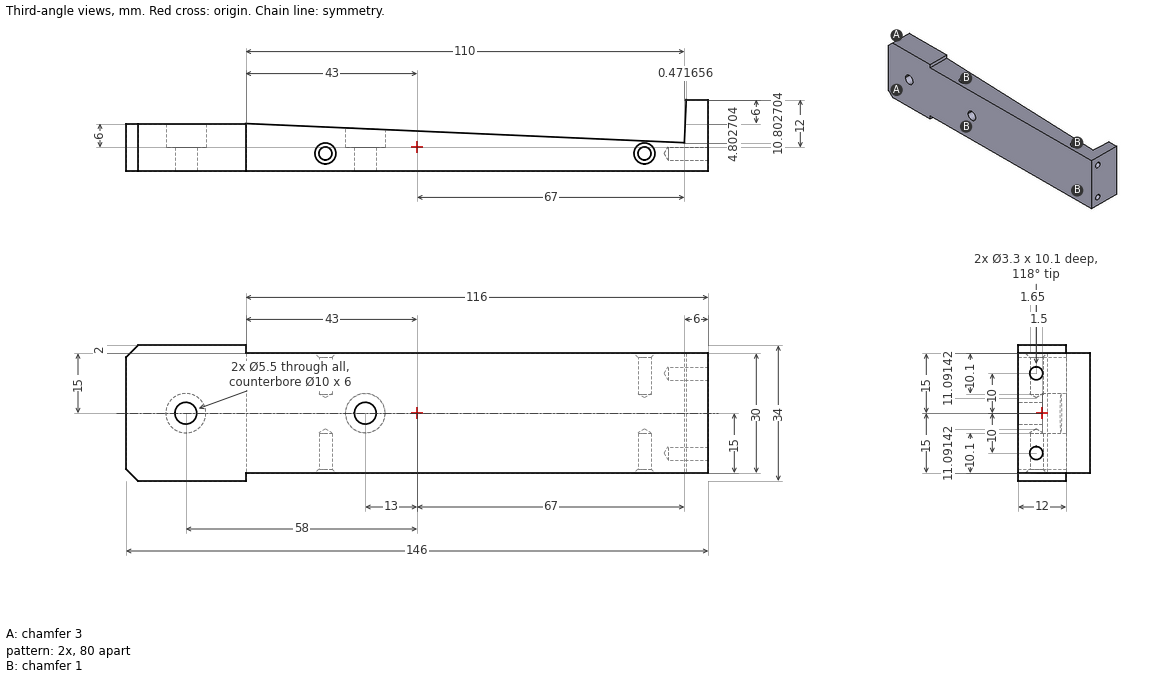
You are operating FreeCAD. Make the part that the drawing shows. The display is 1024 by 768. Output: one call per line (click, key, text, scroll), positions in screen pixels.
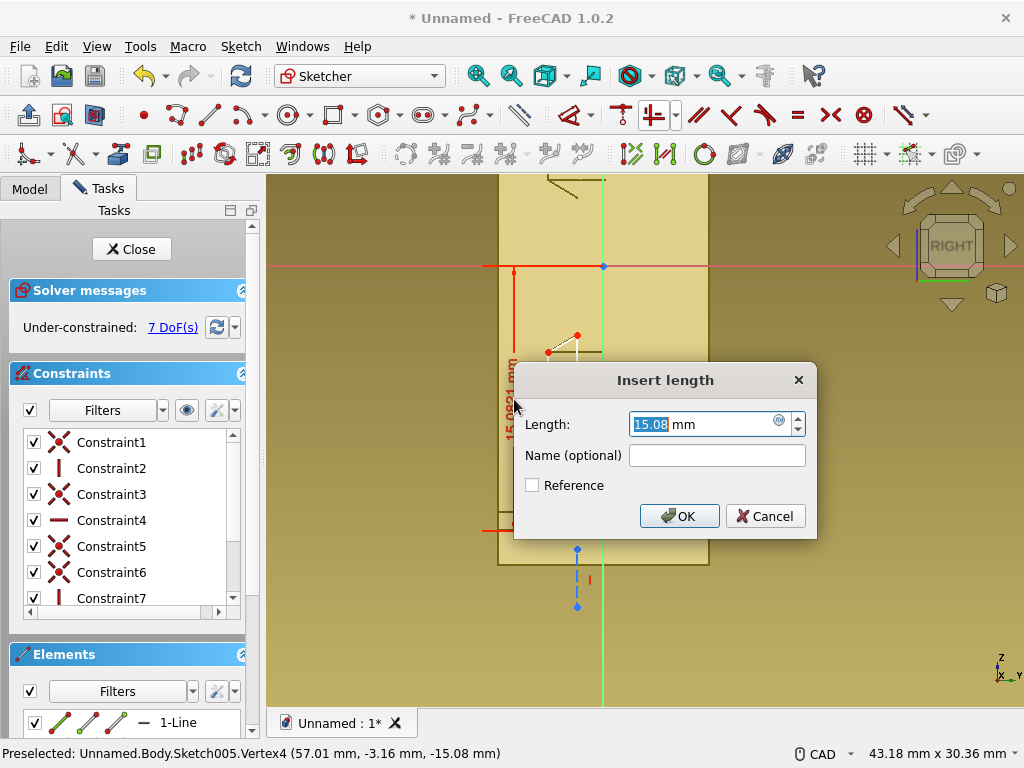
text(15)
key(Return)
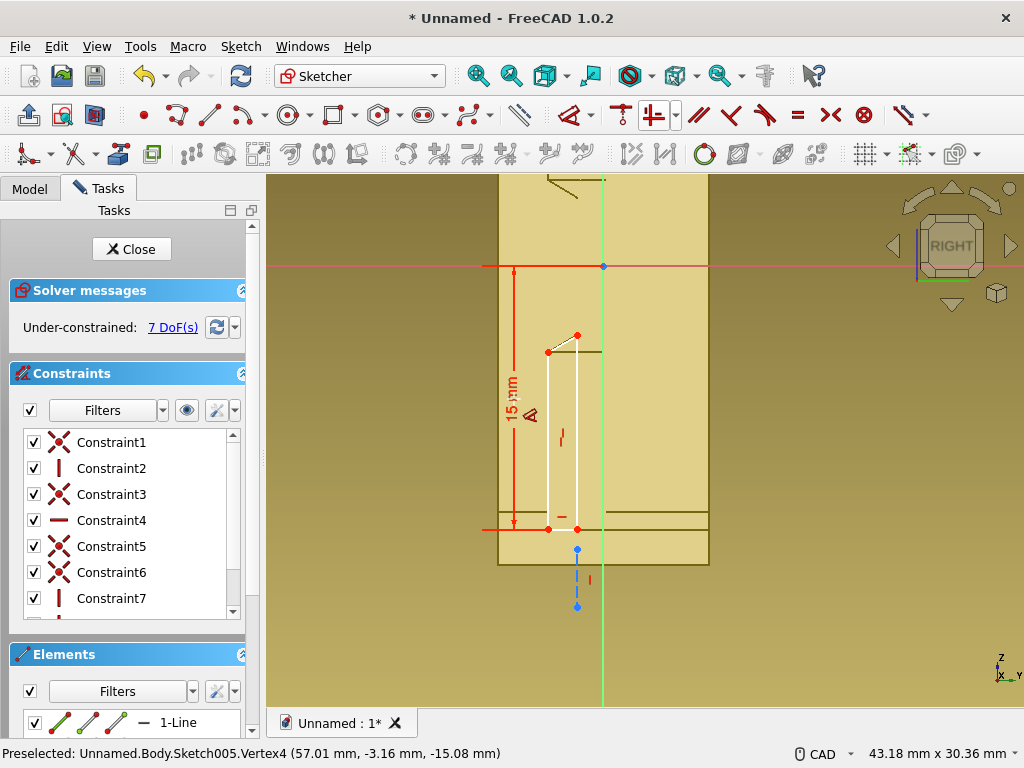
click(548, 406)
click(514, 441)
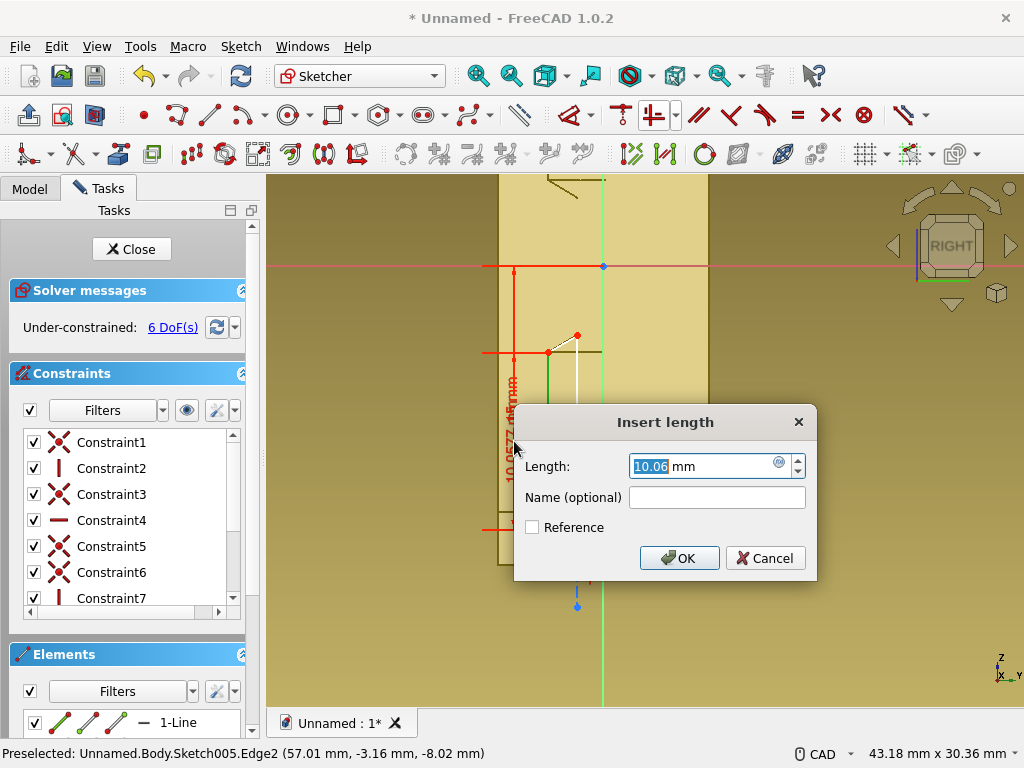
text(10.1)
key(Return)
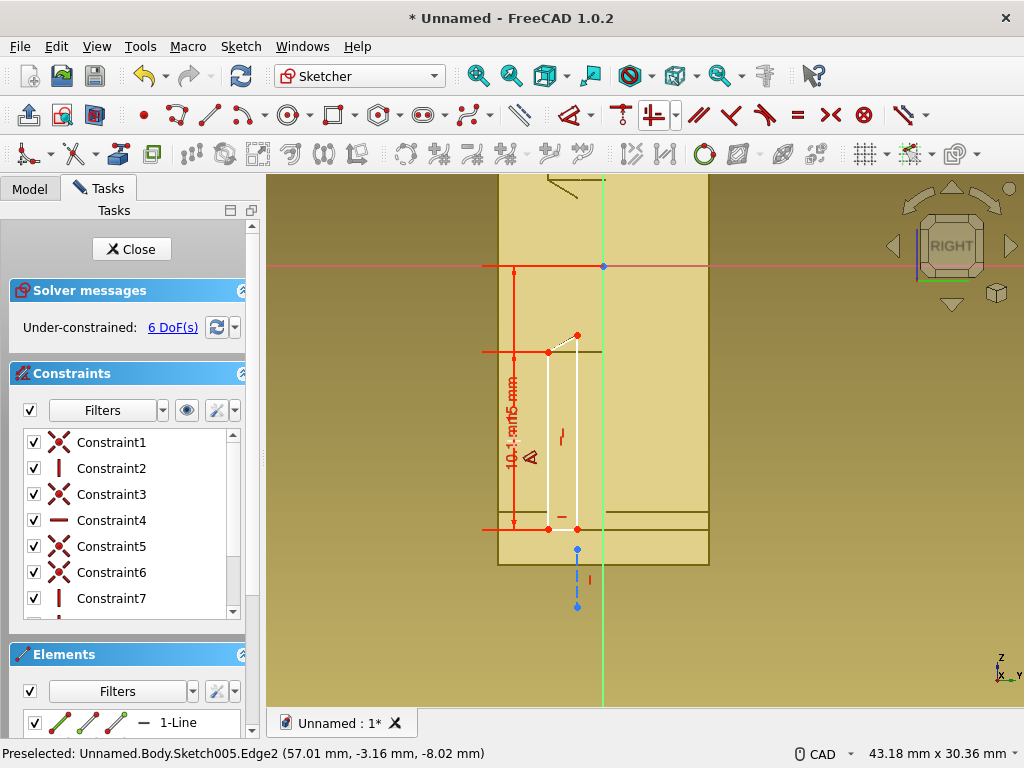
scroll(560, 530, up, 2)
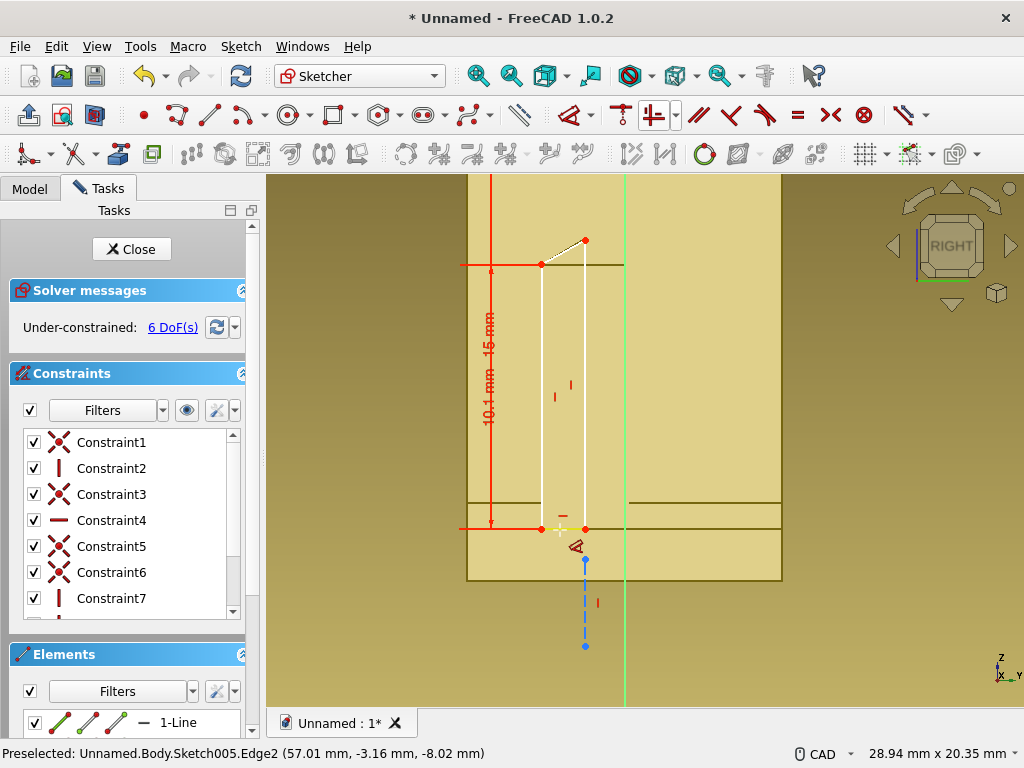
click(559, 529)
click(564, 563)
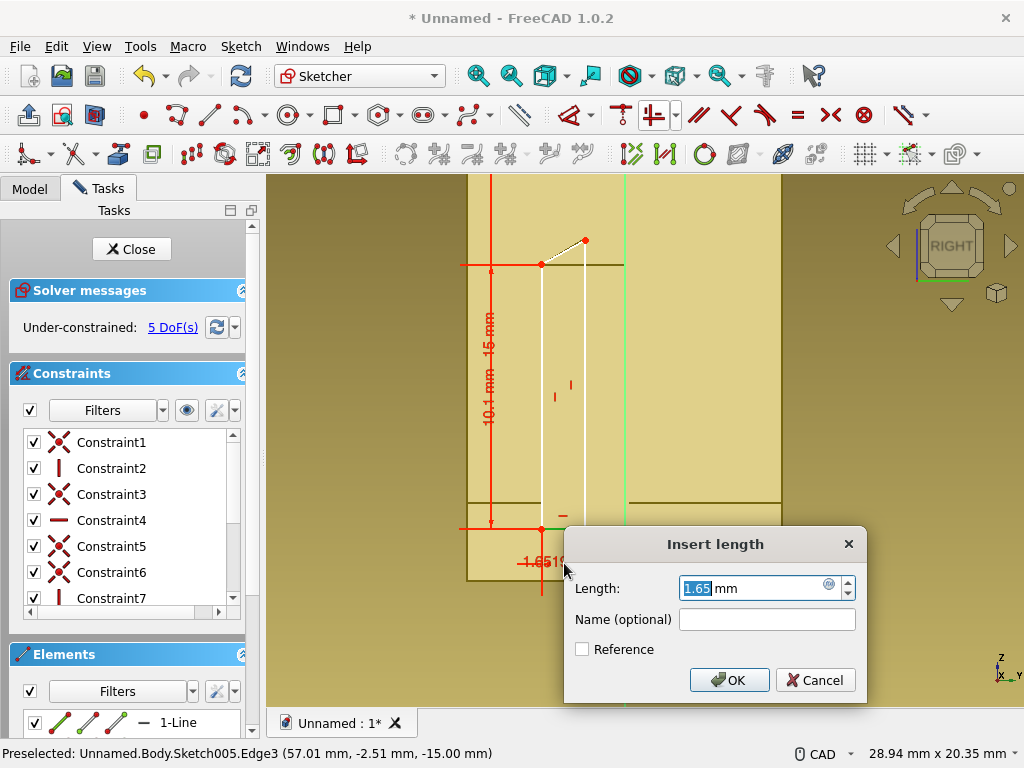
text(1.65)
key(Return)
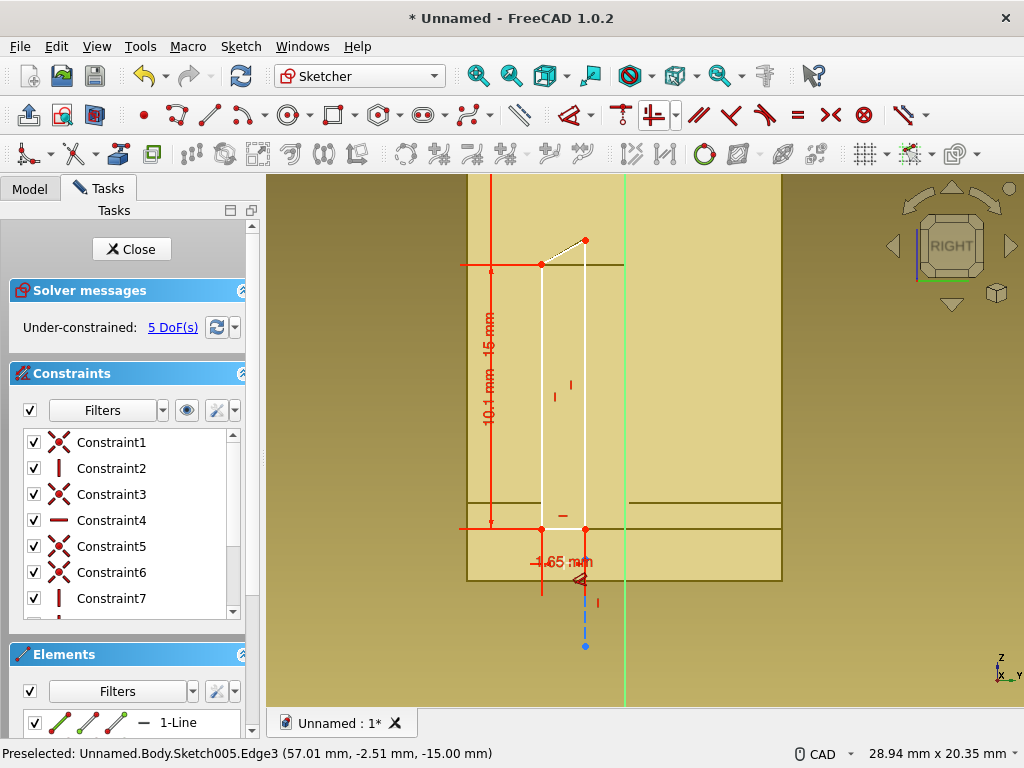
click(585, 240)
click(605, 274)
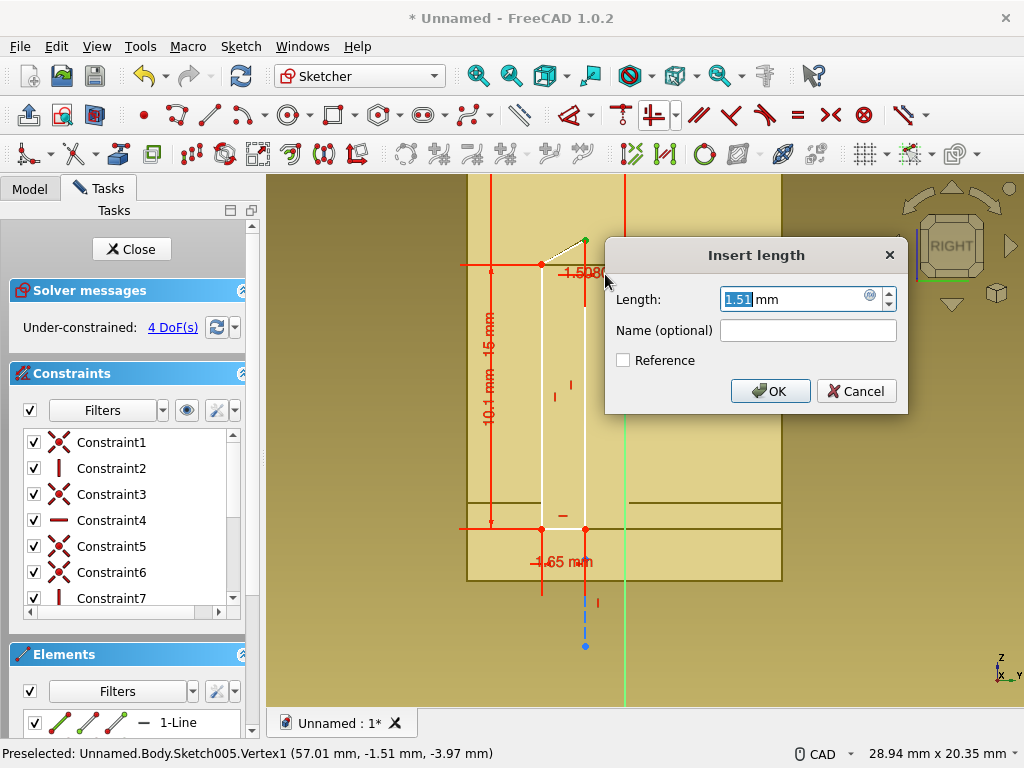
text(1.5)
key(Return)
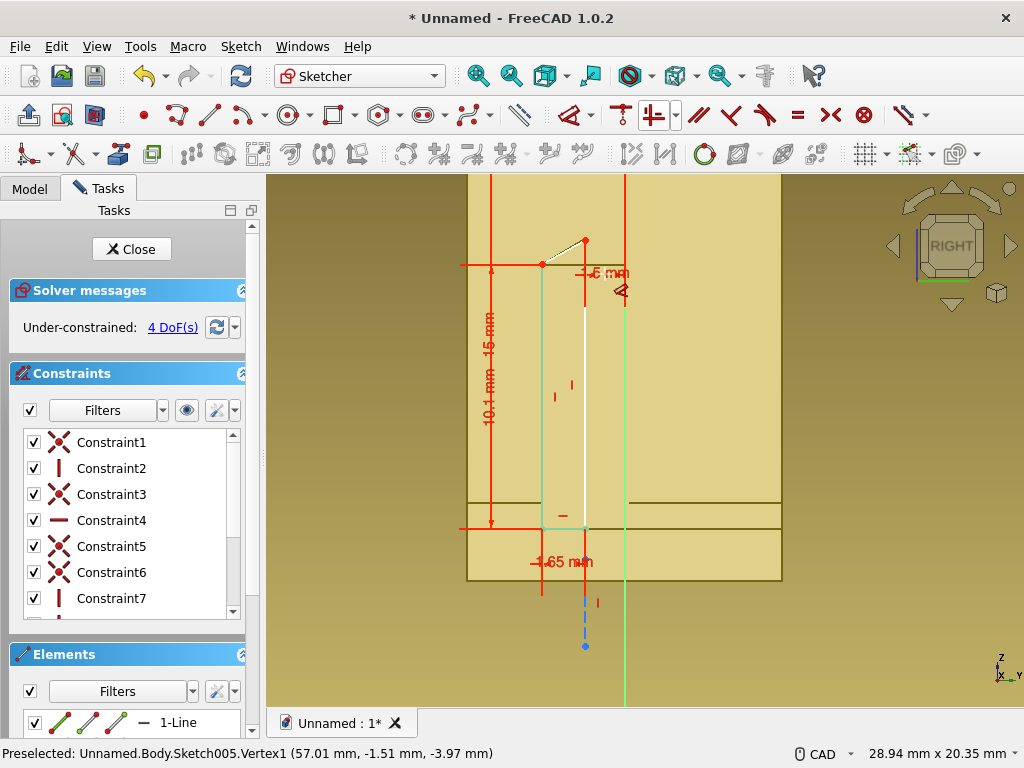
click(585, 560)
click(605, 594)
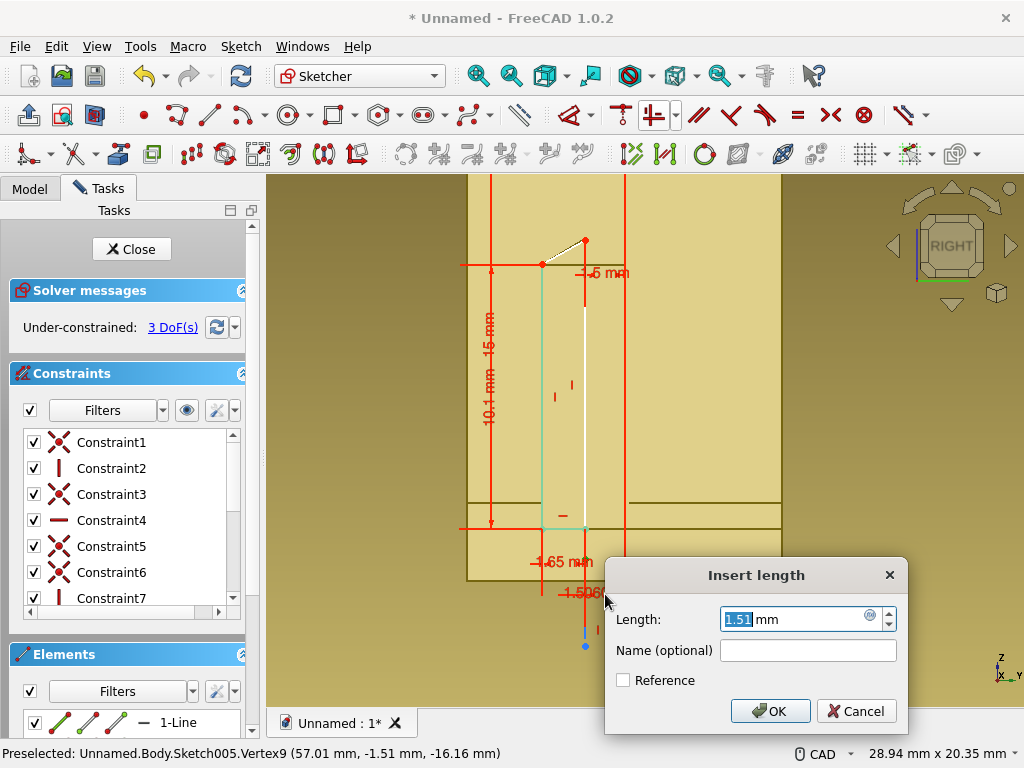
text(1.5)
key(Return)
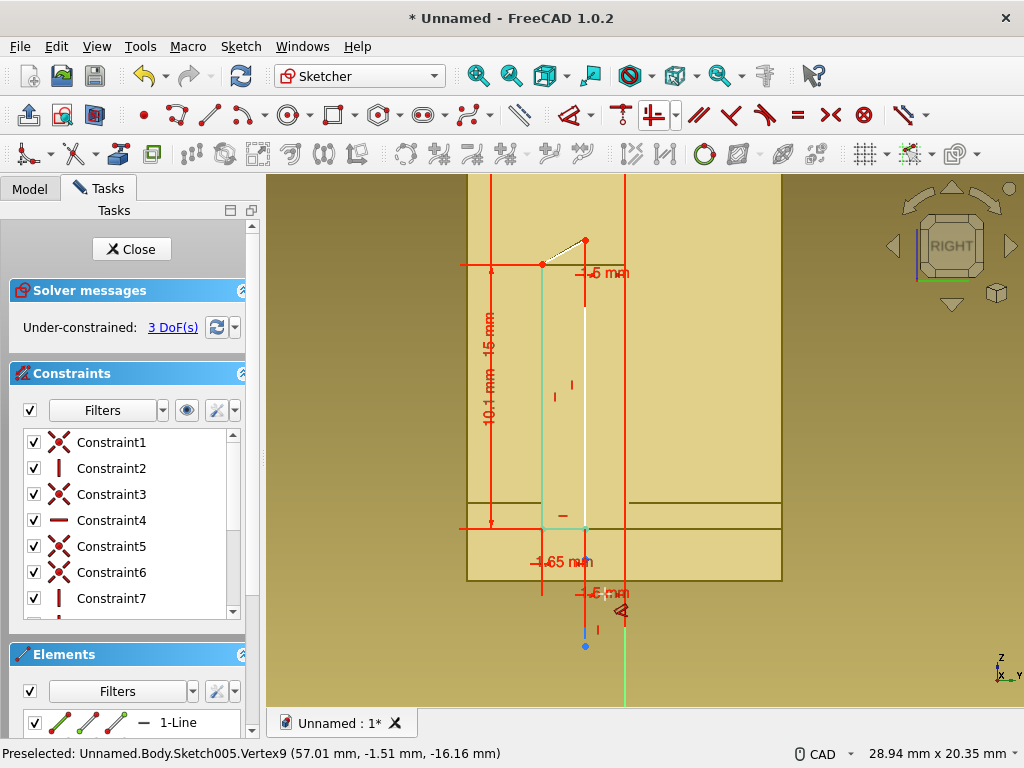
click(585, 442)
click(643, 385)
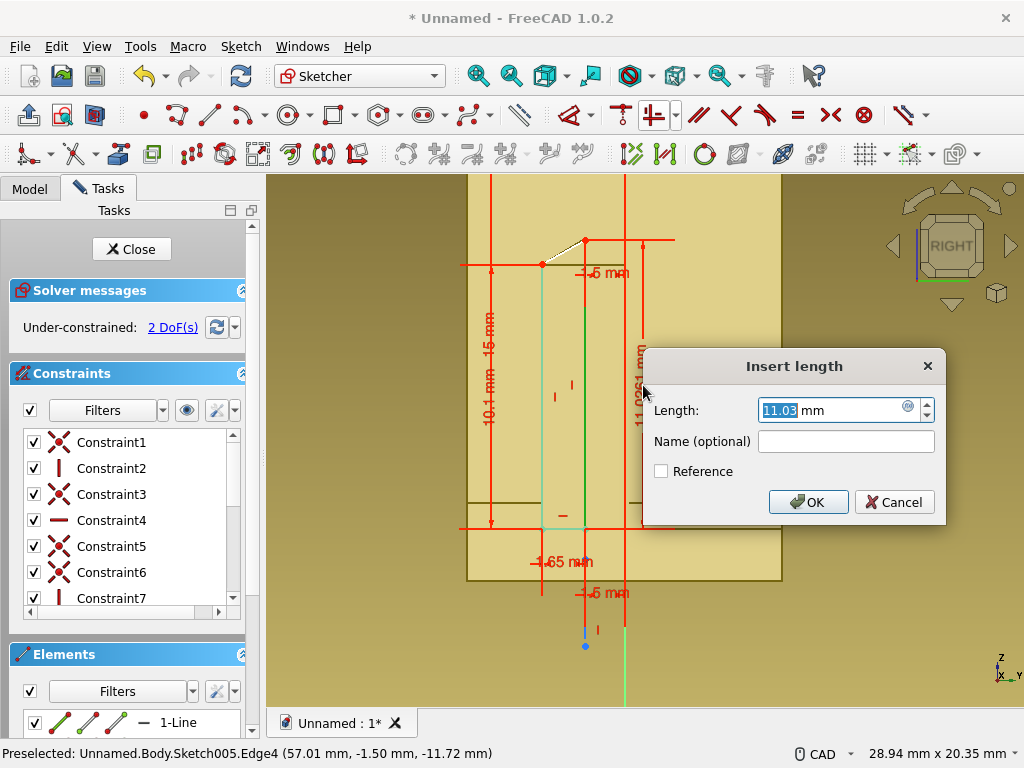
text(11.09142)
key(Return)
key(Escape)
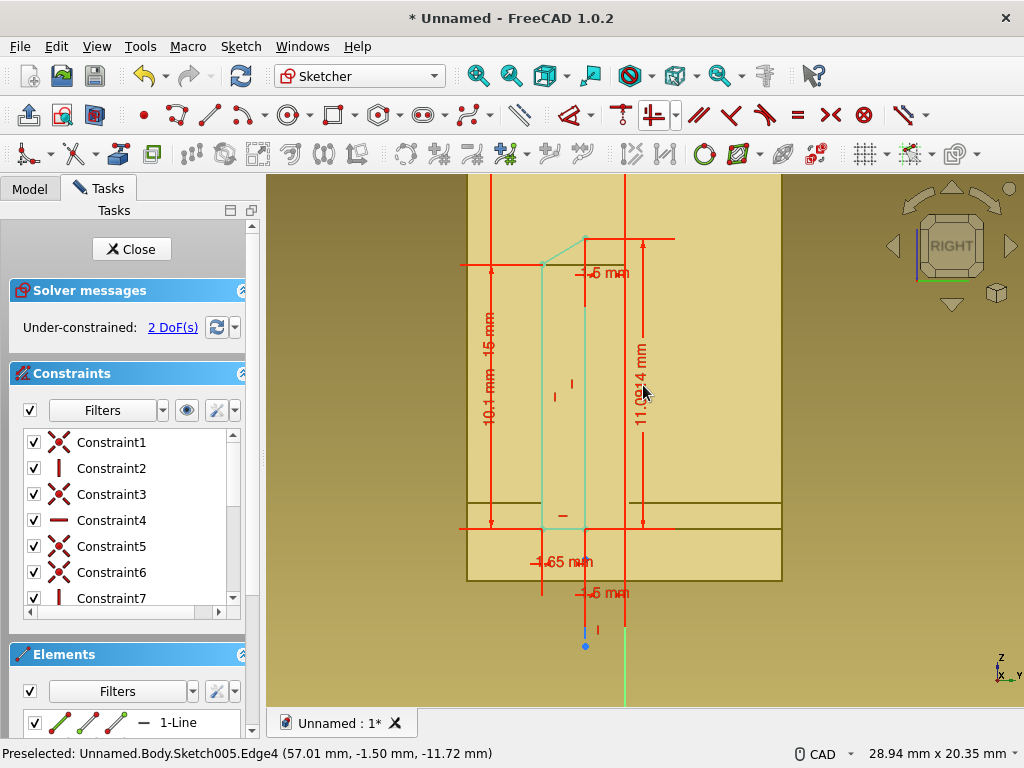
click(132, 249)